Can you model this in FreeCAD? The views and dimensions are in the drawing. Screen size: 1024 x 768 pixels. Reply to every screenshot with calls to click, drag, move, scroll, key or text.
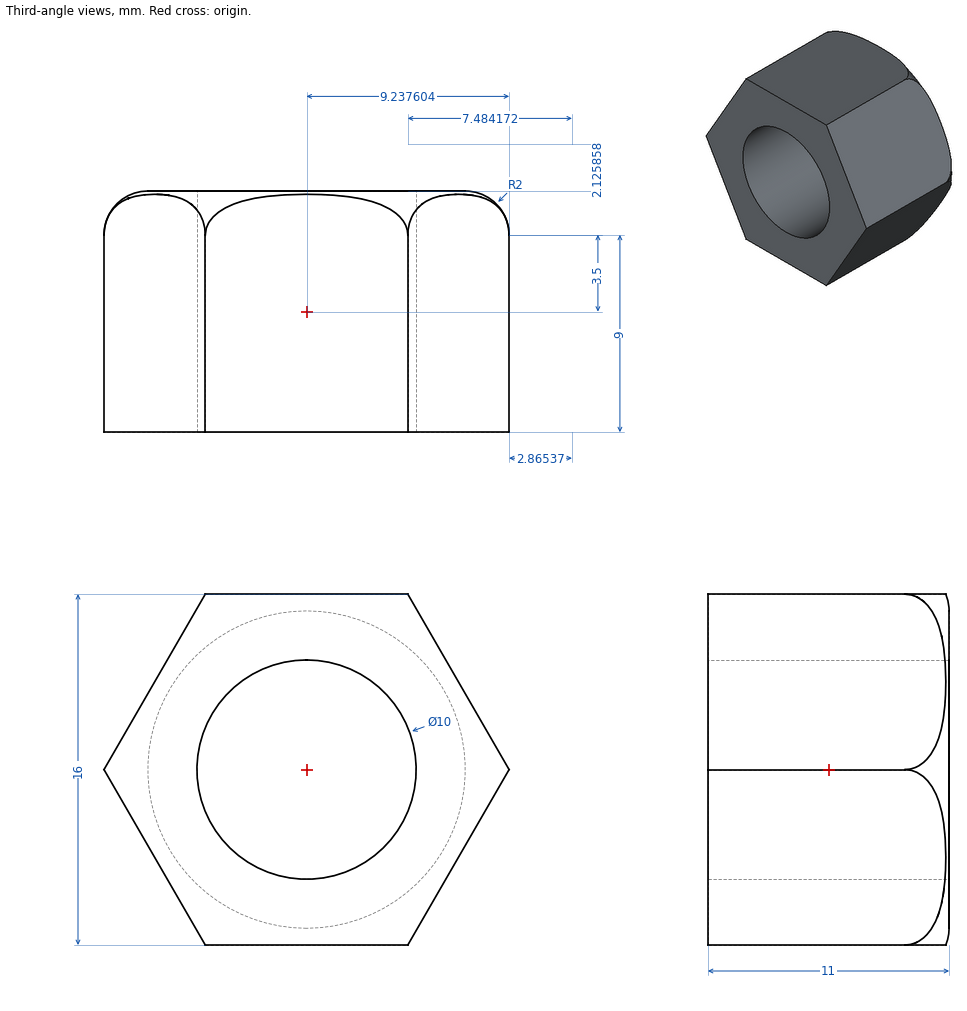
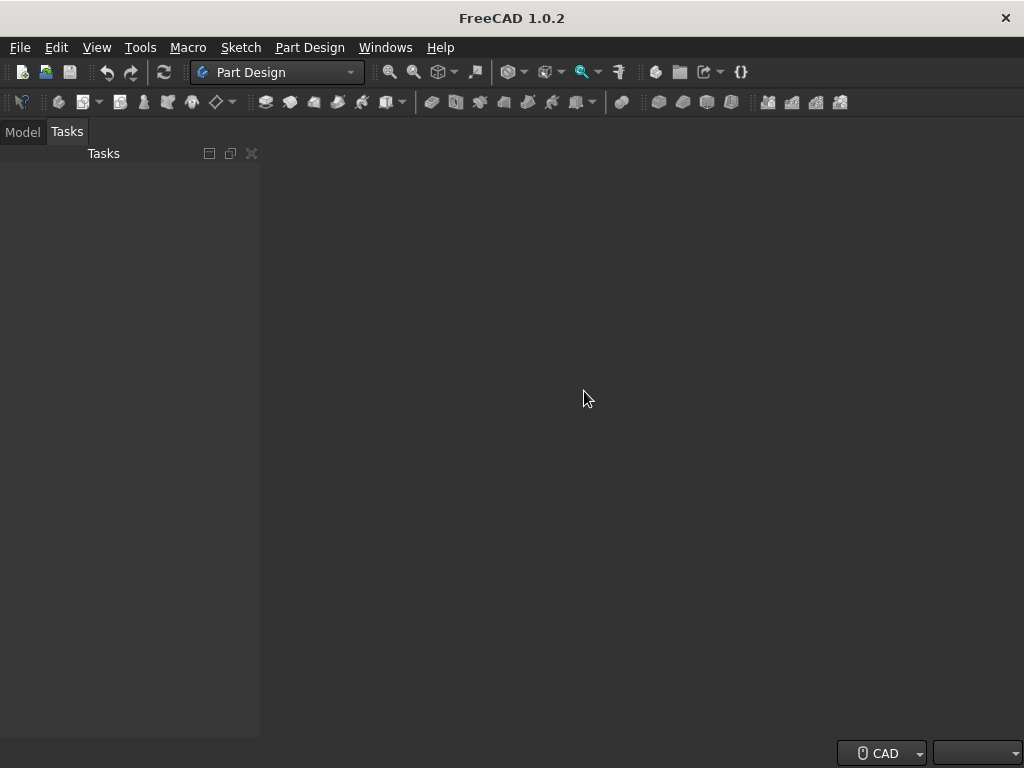
click(22, 72)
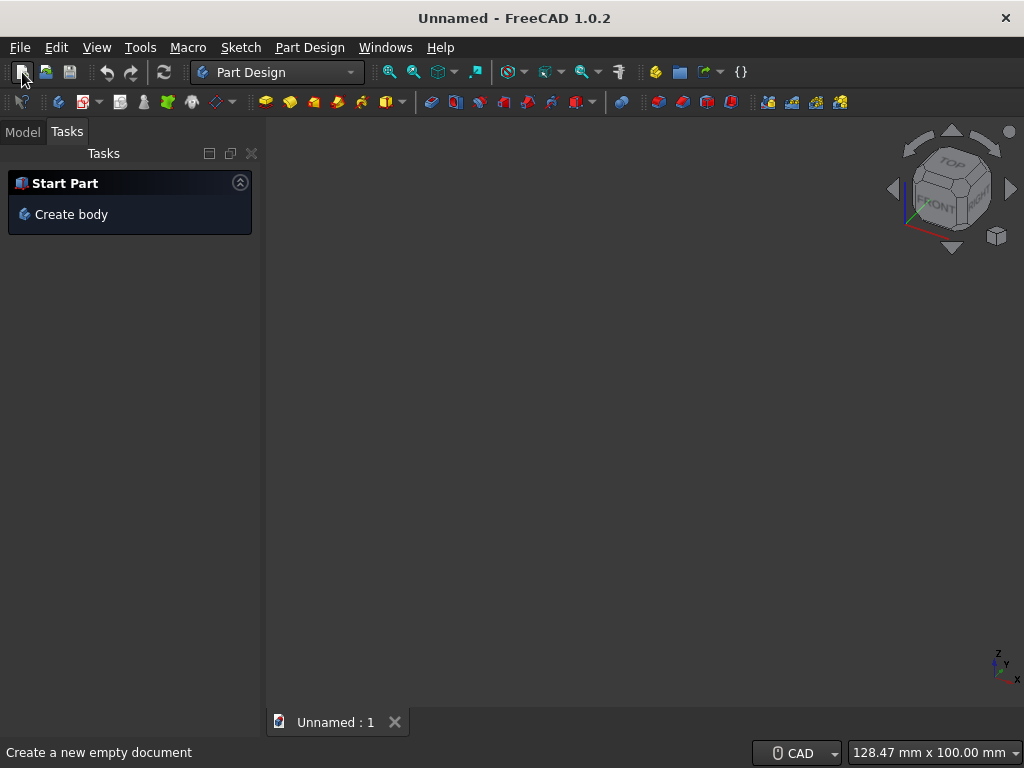
click(84, 102)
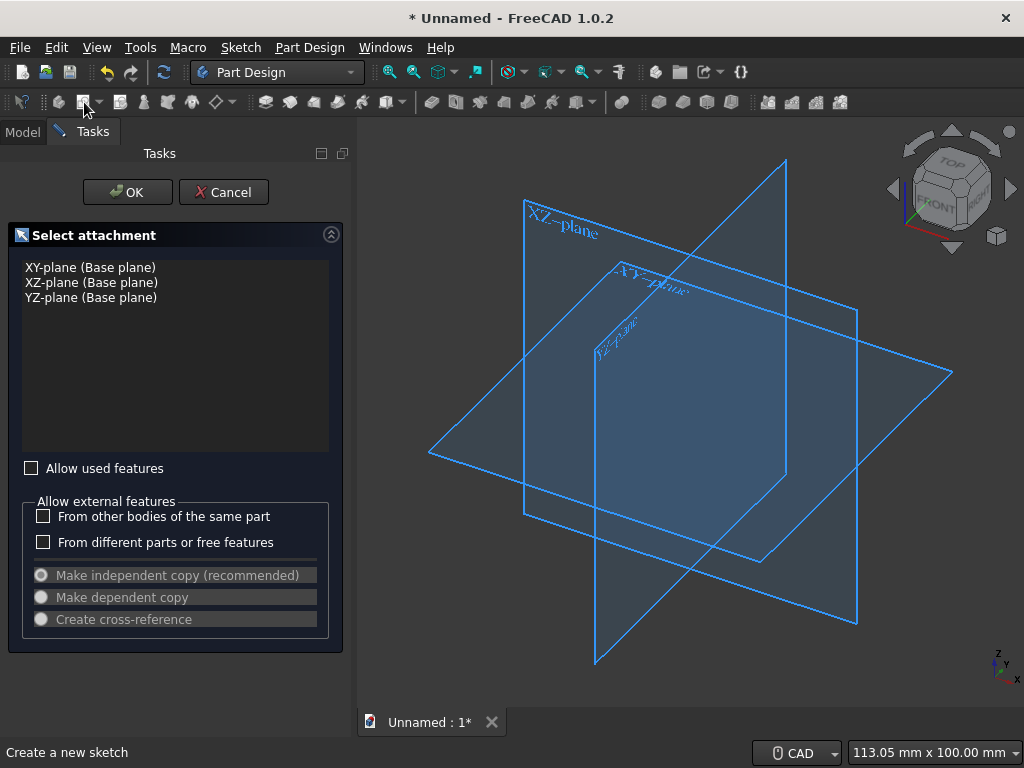
click(82, 282)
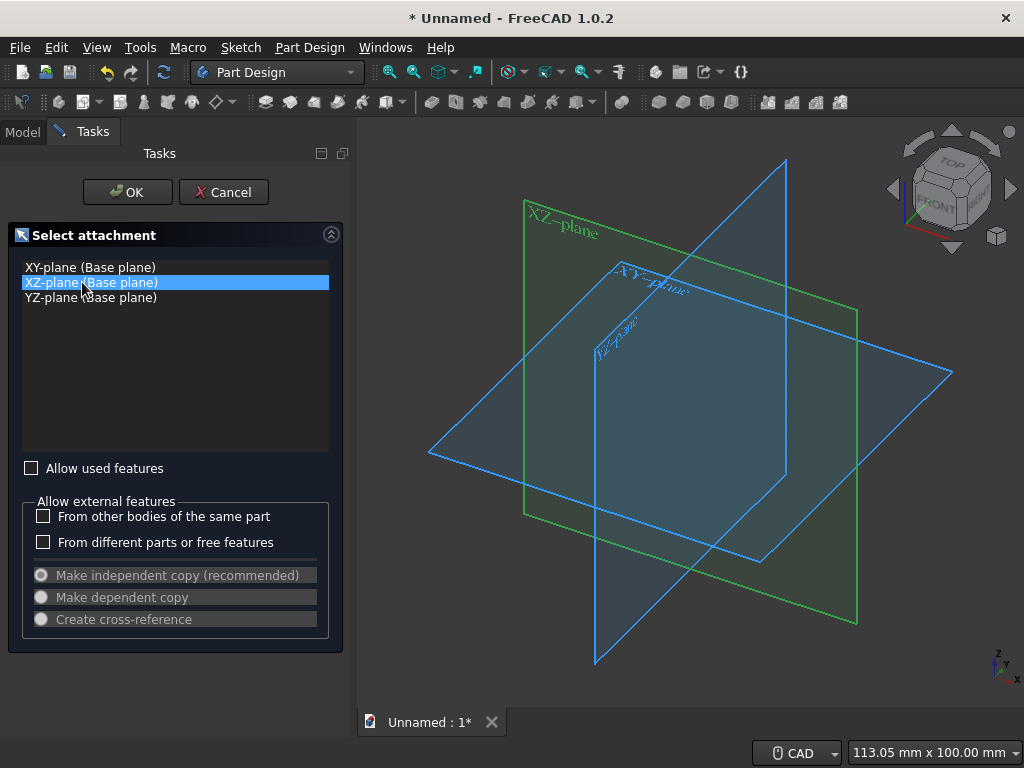
click(128, 192)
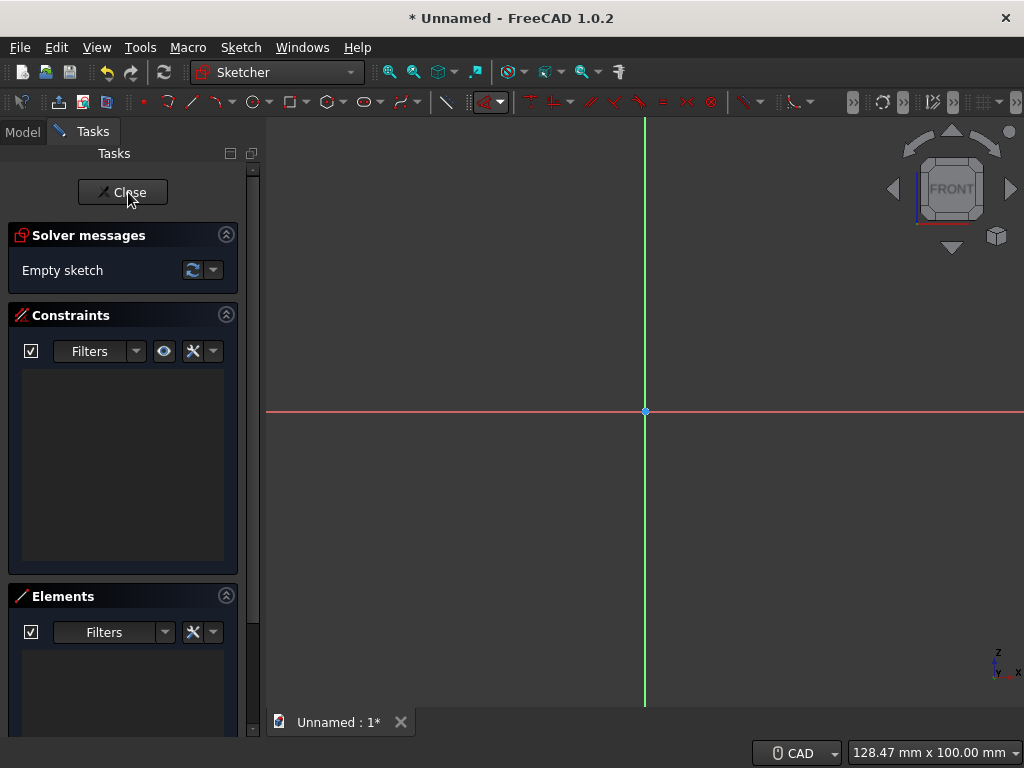
scroll(675, 412, up, 6)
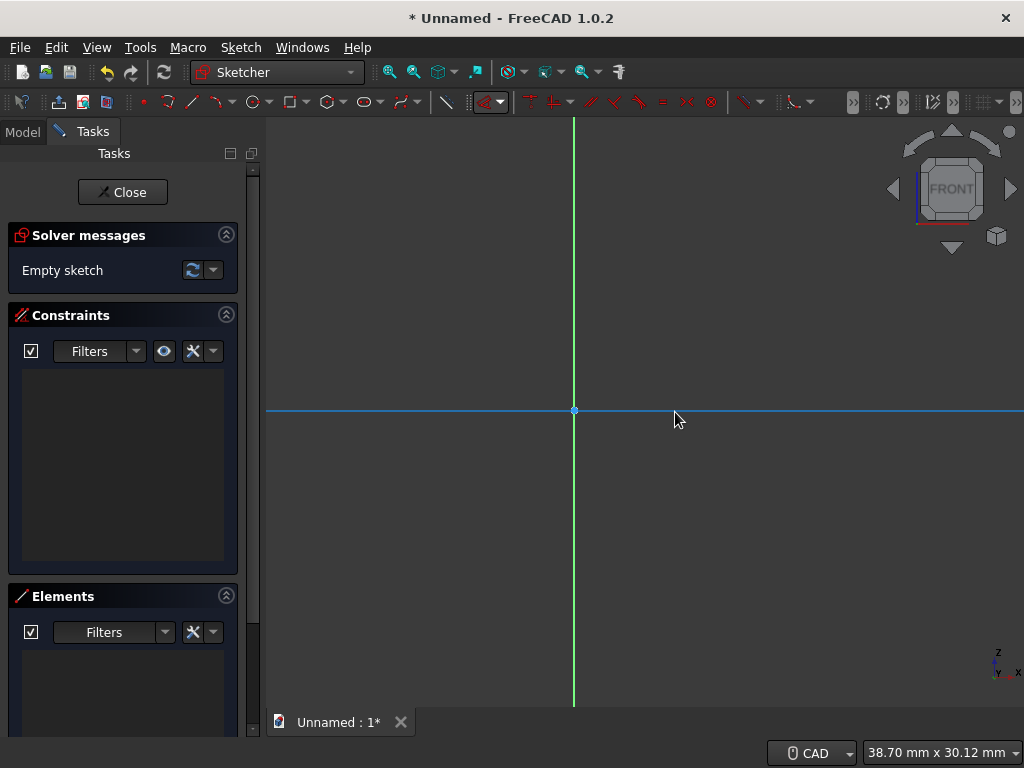
key(g)
key(p)
key(6)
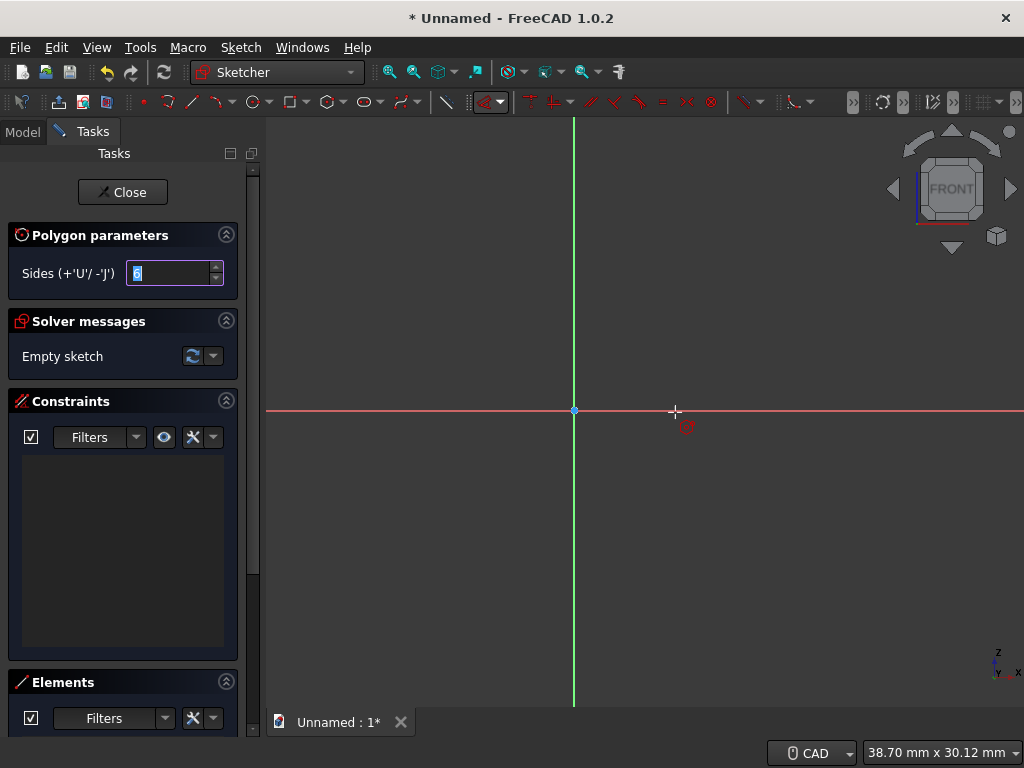
click(574, 411)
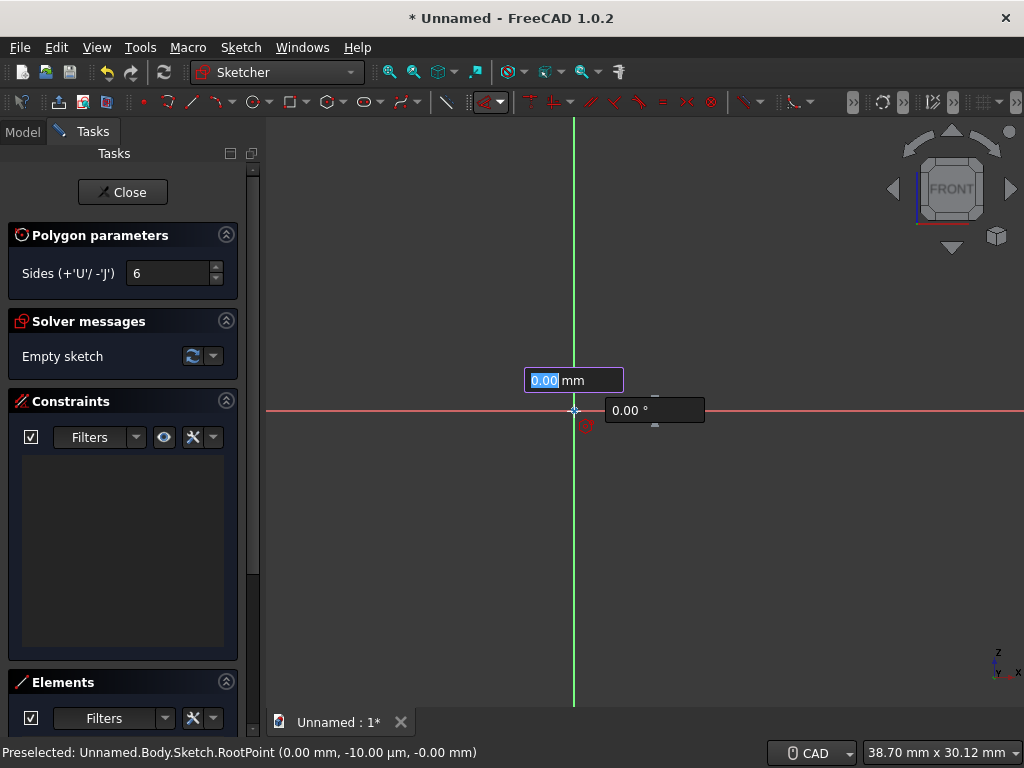
click(755, 411)
right_click(755, 411)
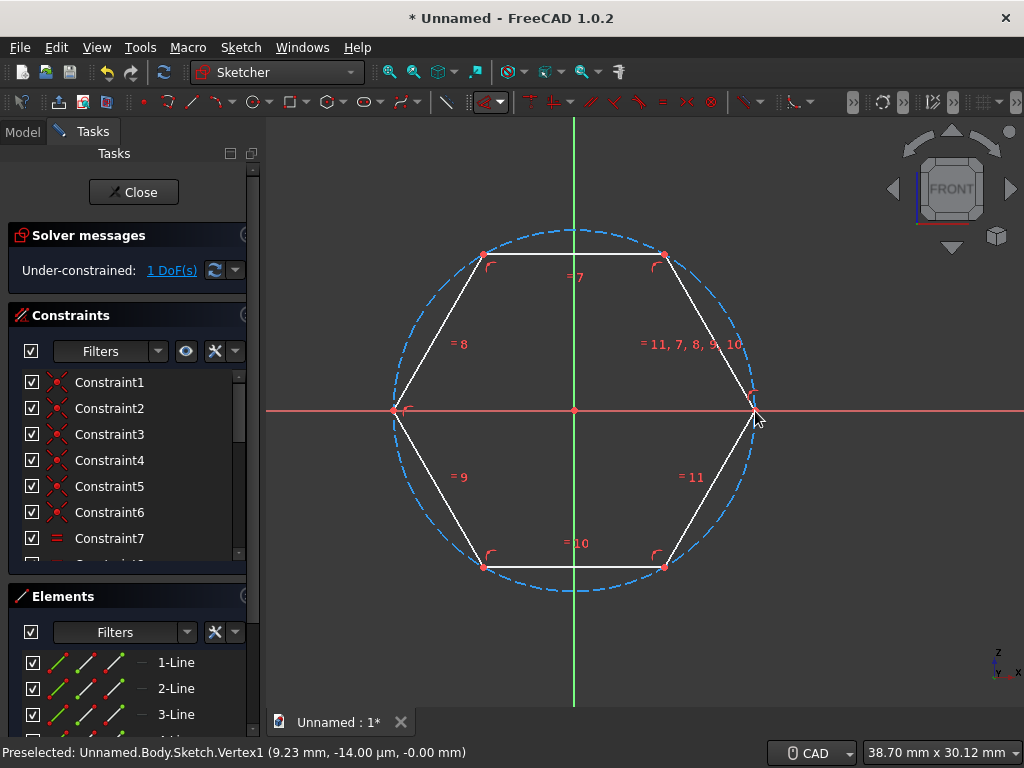
click(484, 567)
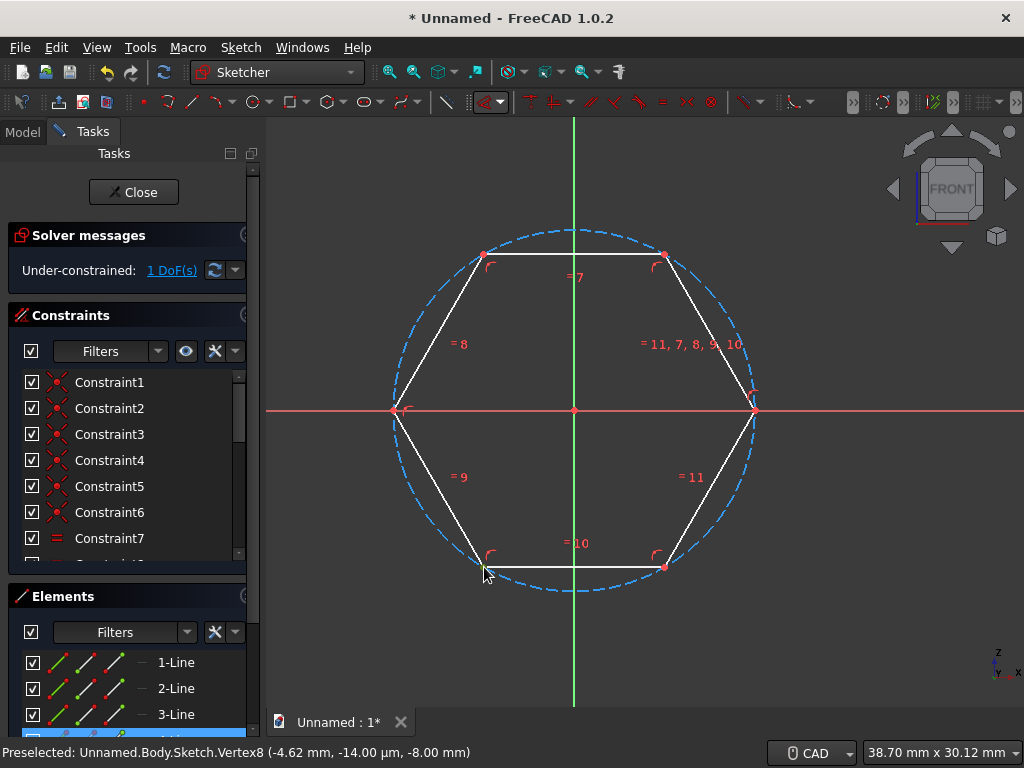
click(665, 254)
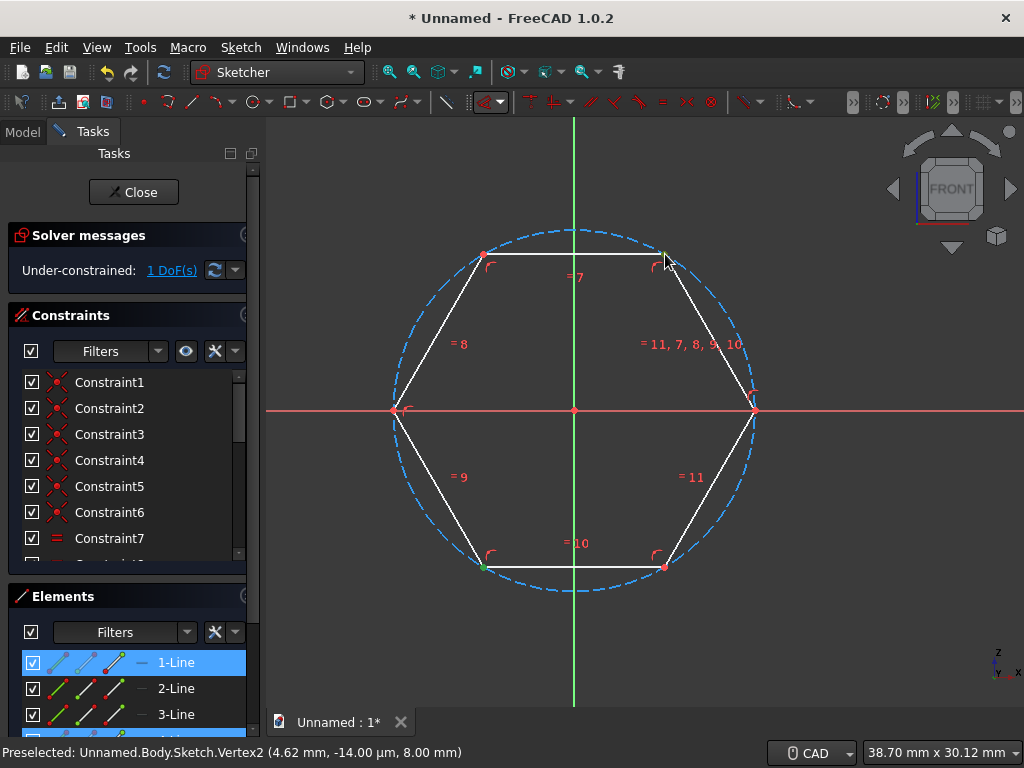
key(i)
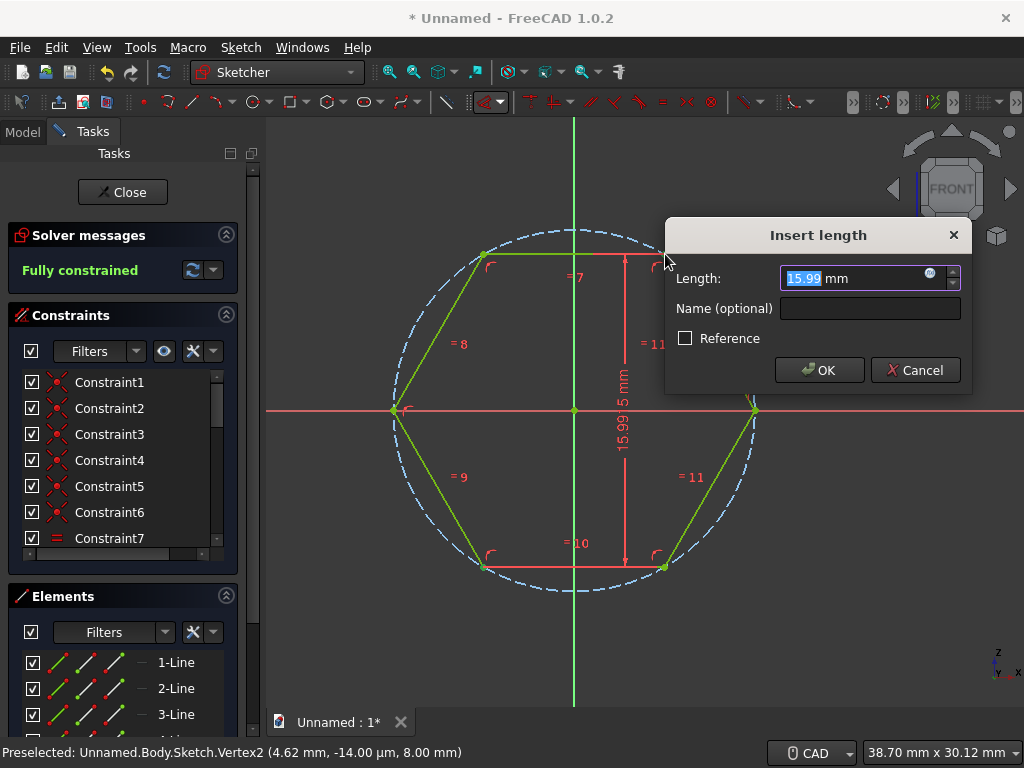
text(16)
key(Return)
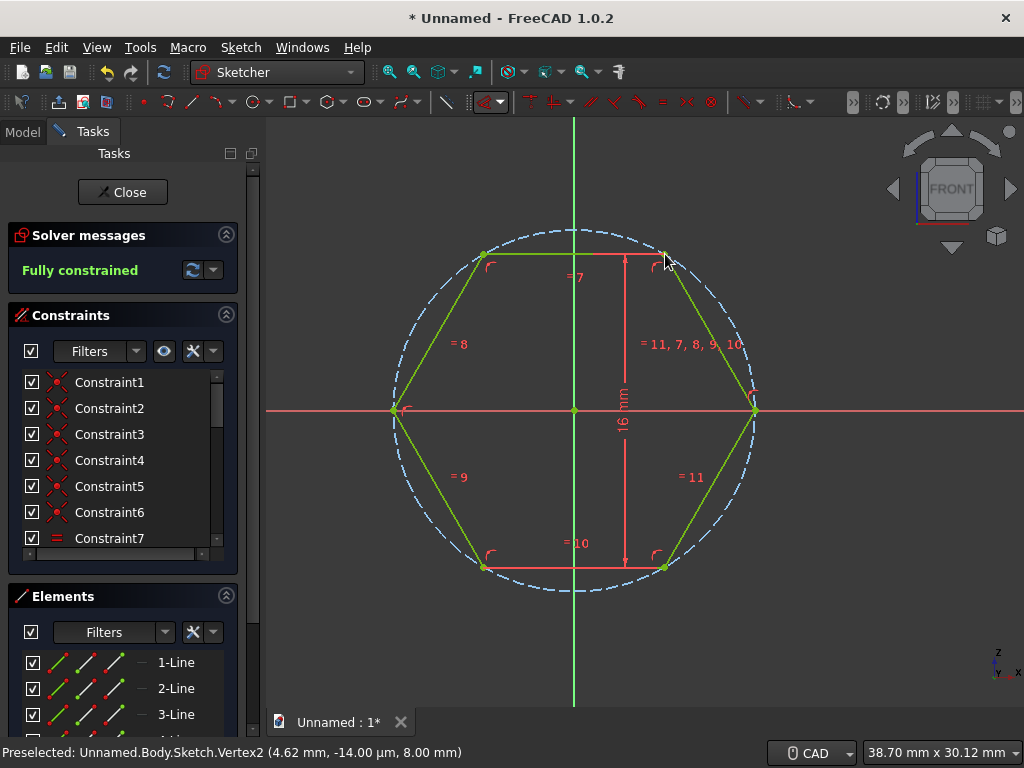
click(123, 192)